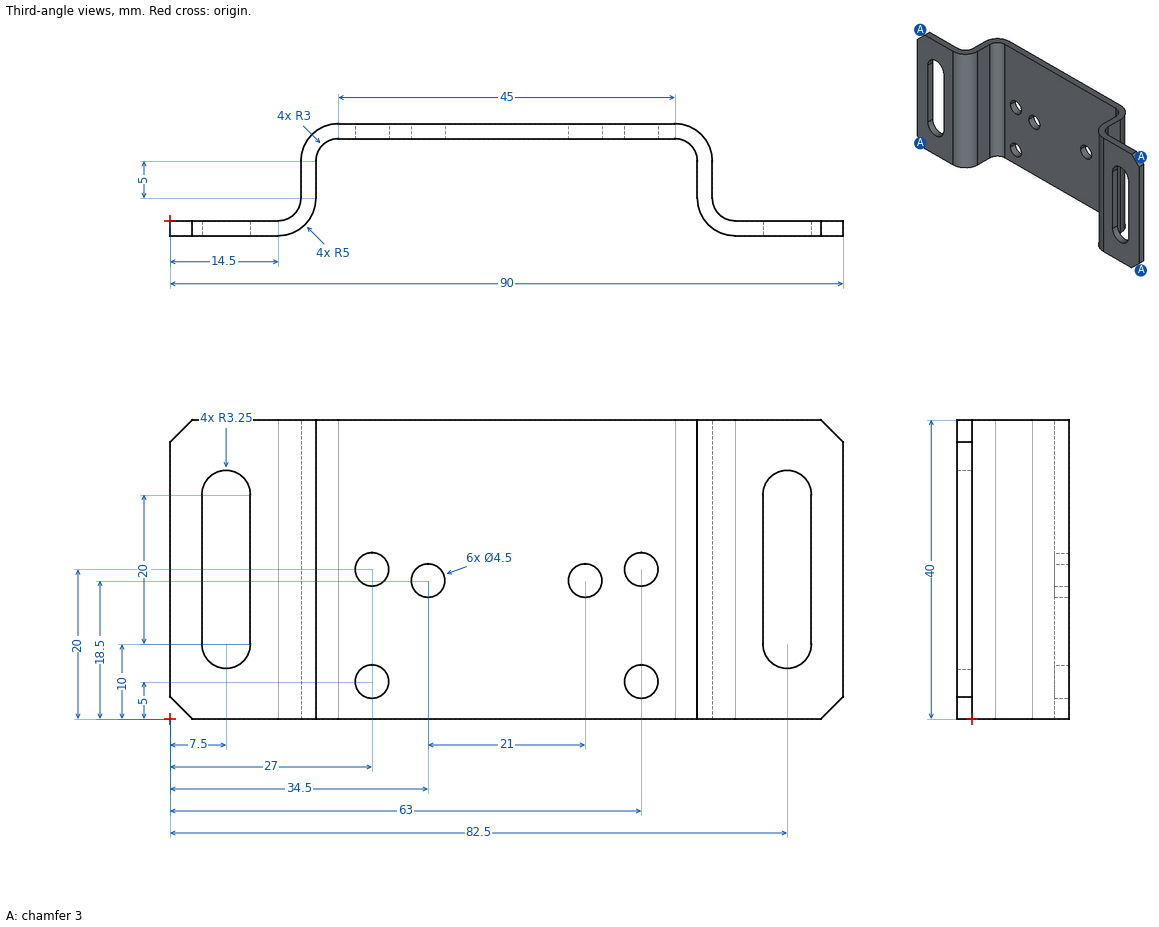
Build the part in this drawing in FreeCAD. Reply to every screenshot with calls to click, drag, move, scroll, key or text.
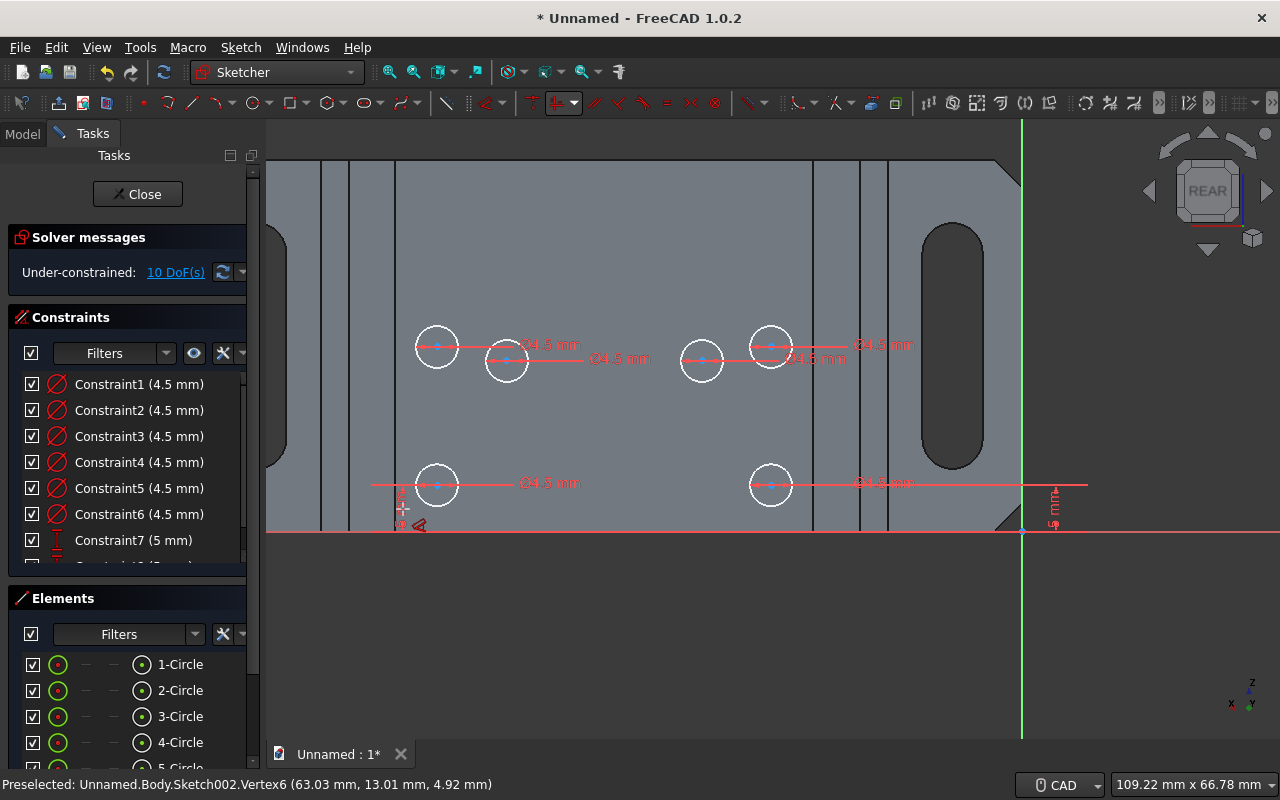
click(771, 347)
click(897, 566)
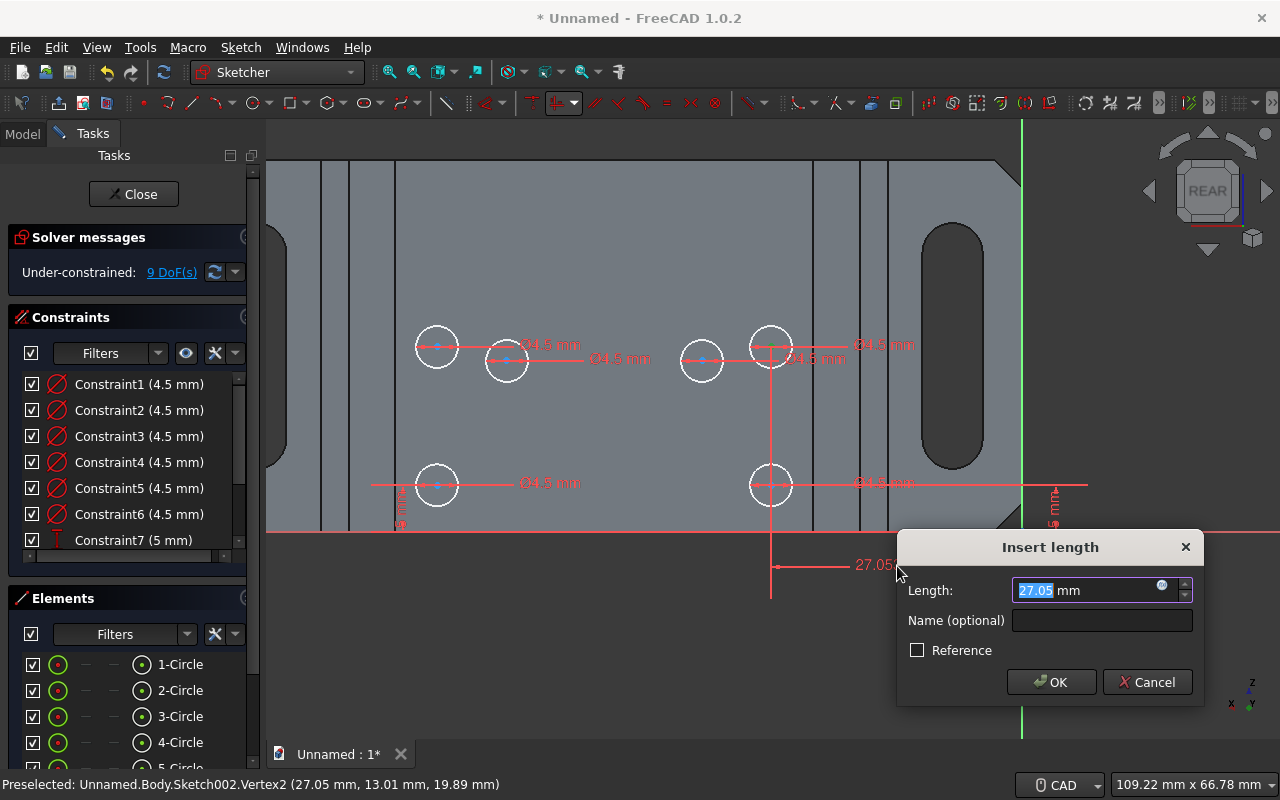
text(27)
key(Return)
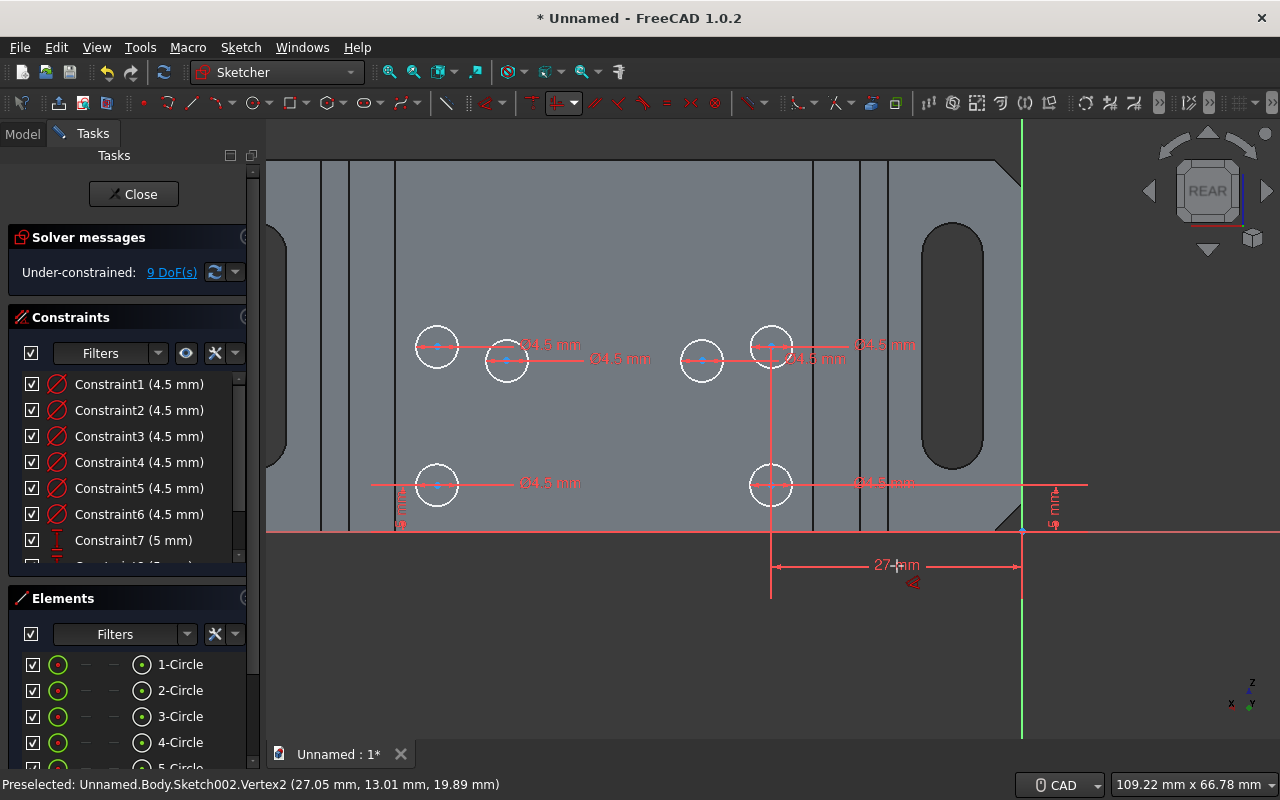
click(771, 347)
click(1056, 439)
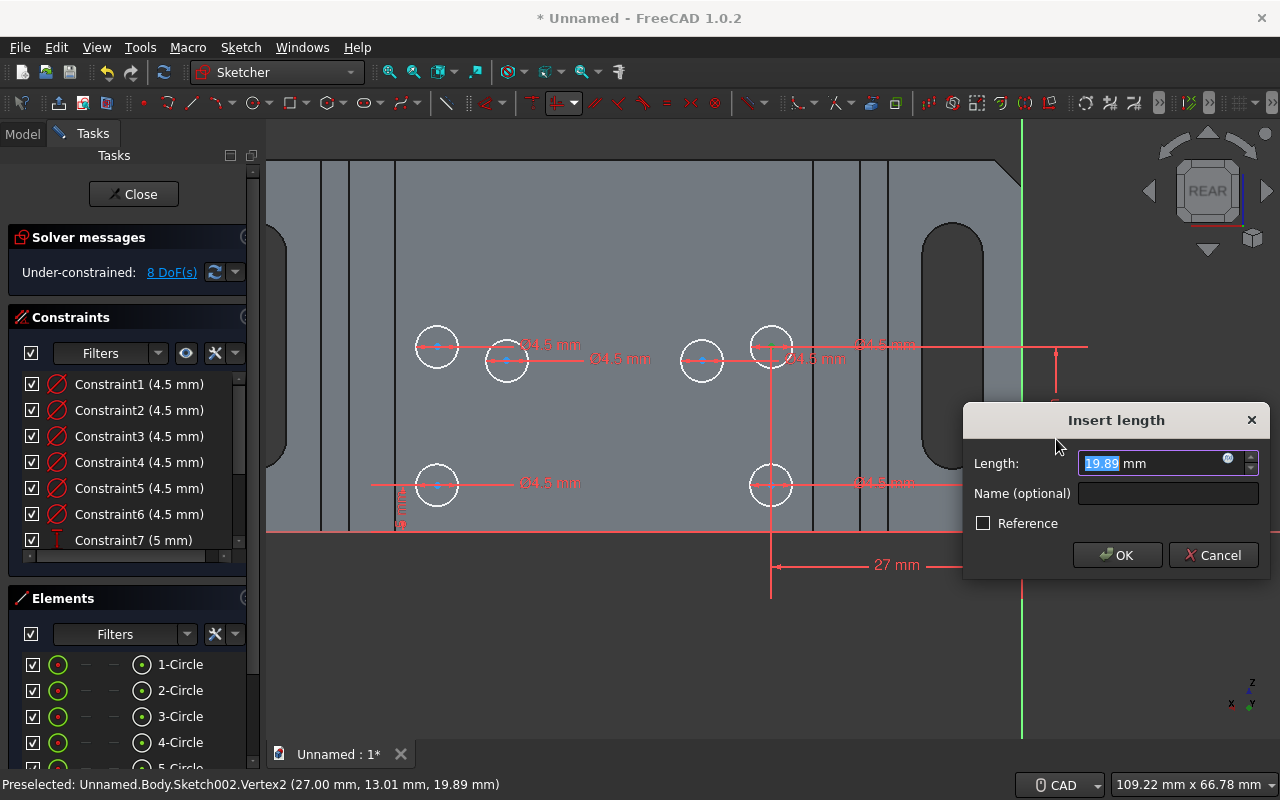
text(20)
key(Return)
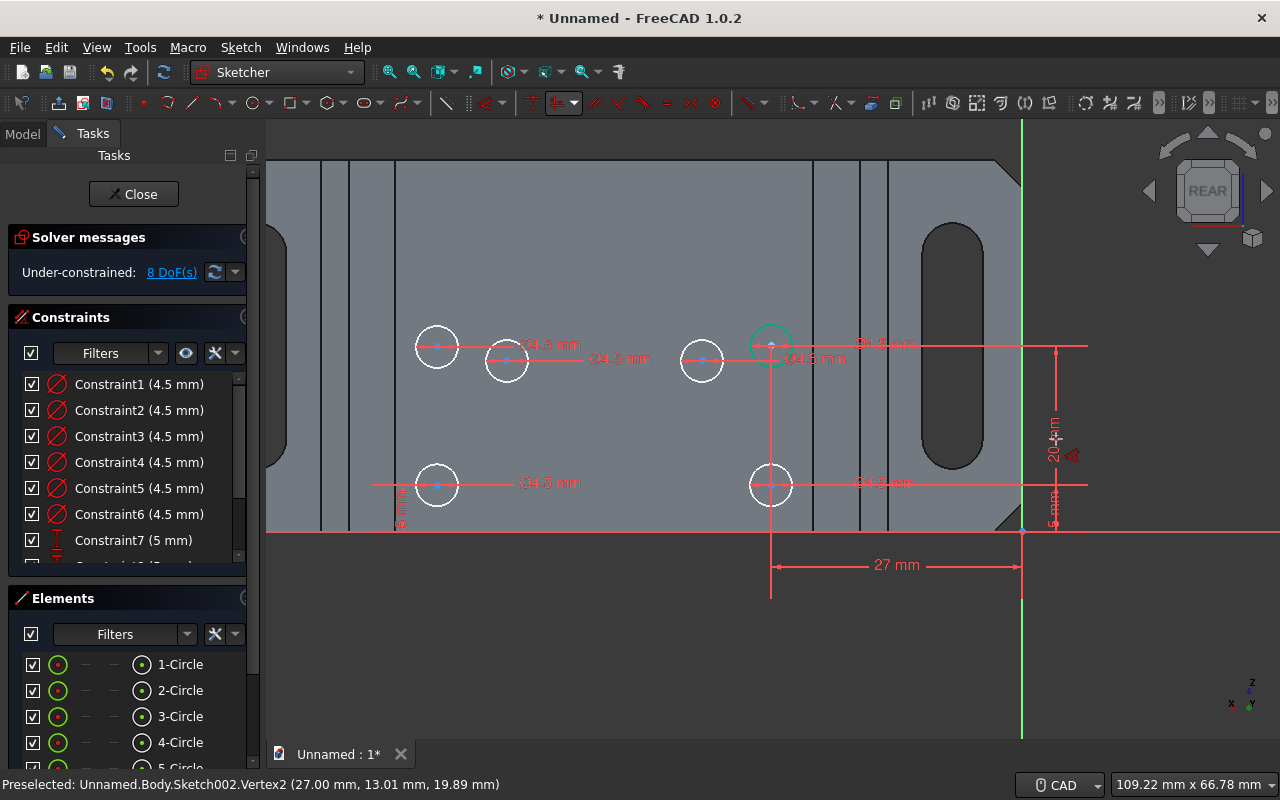
click(437, 347)
click(730, 566)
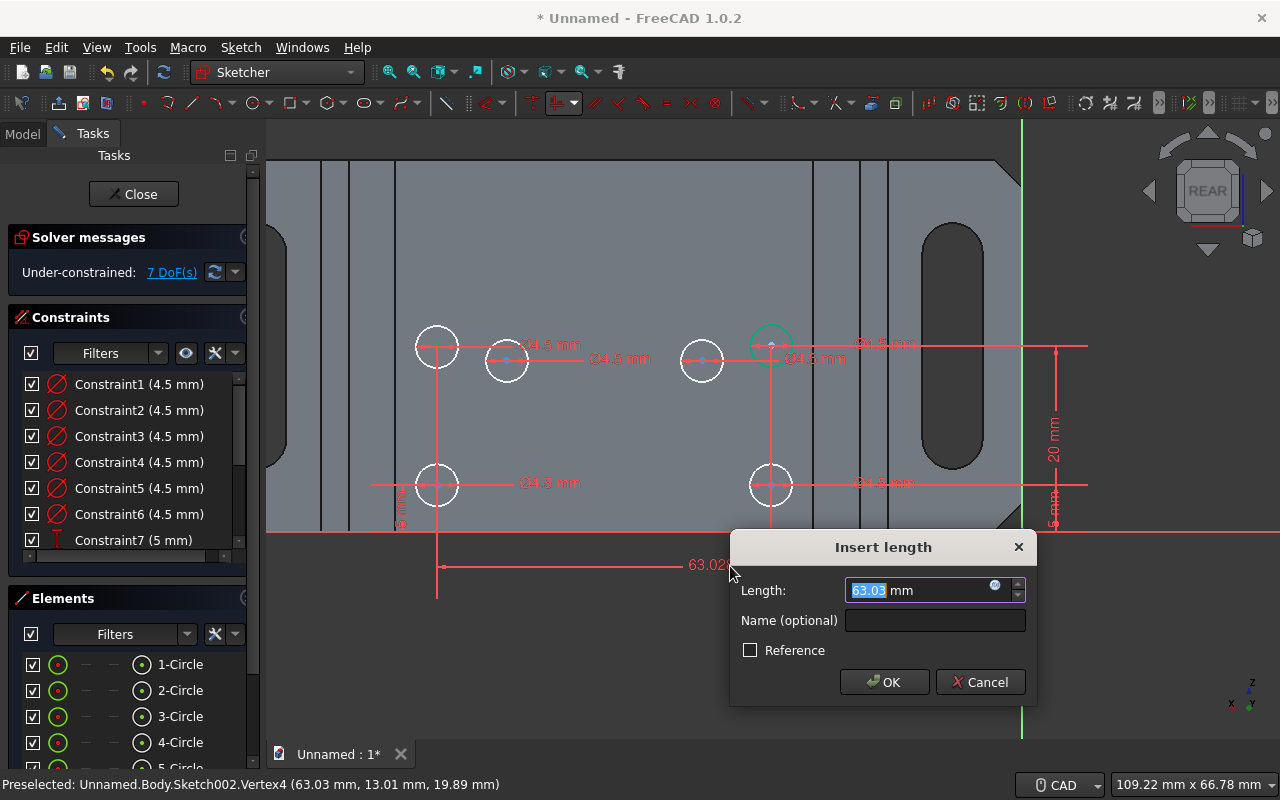
text(63)
key(Return)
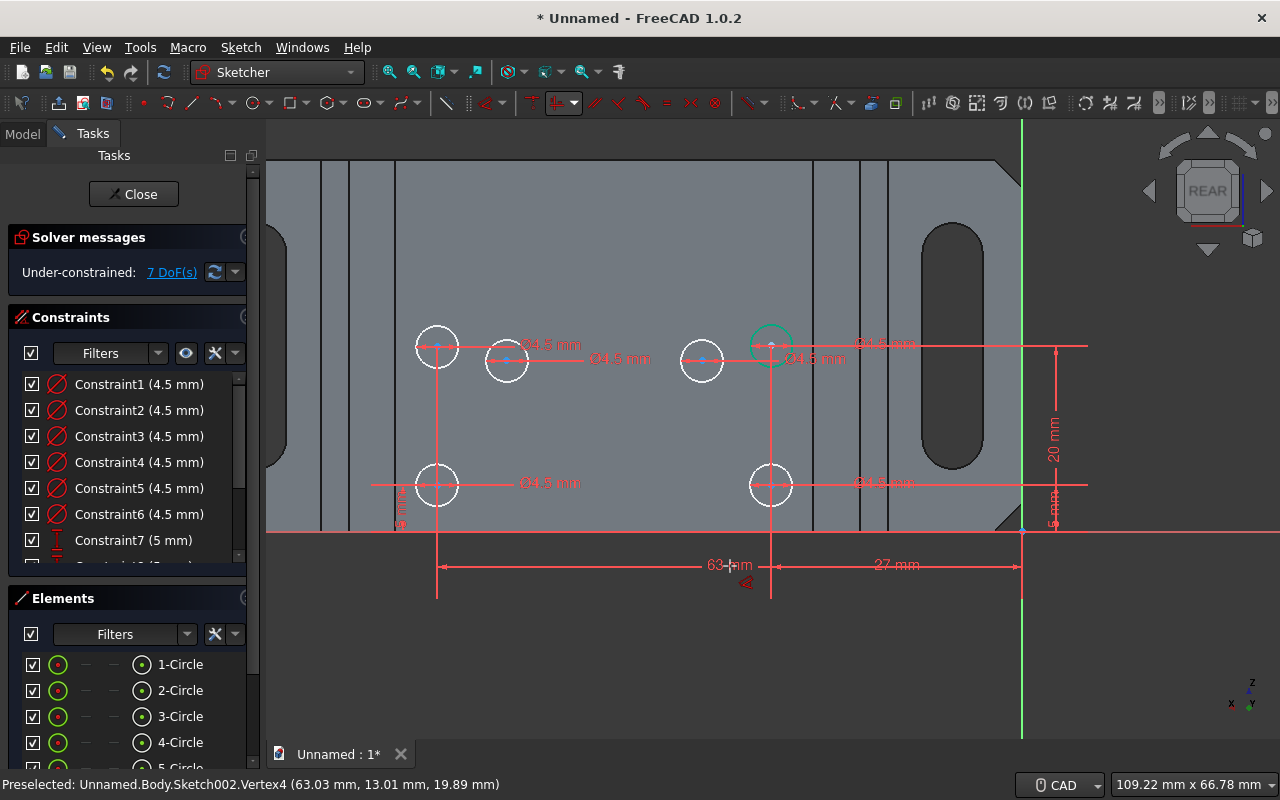
click(437, 347)
click(1056, 397)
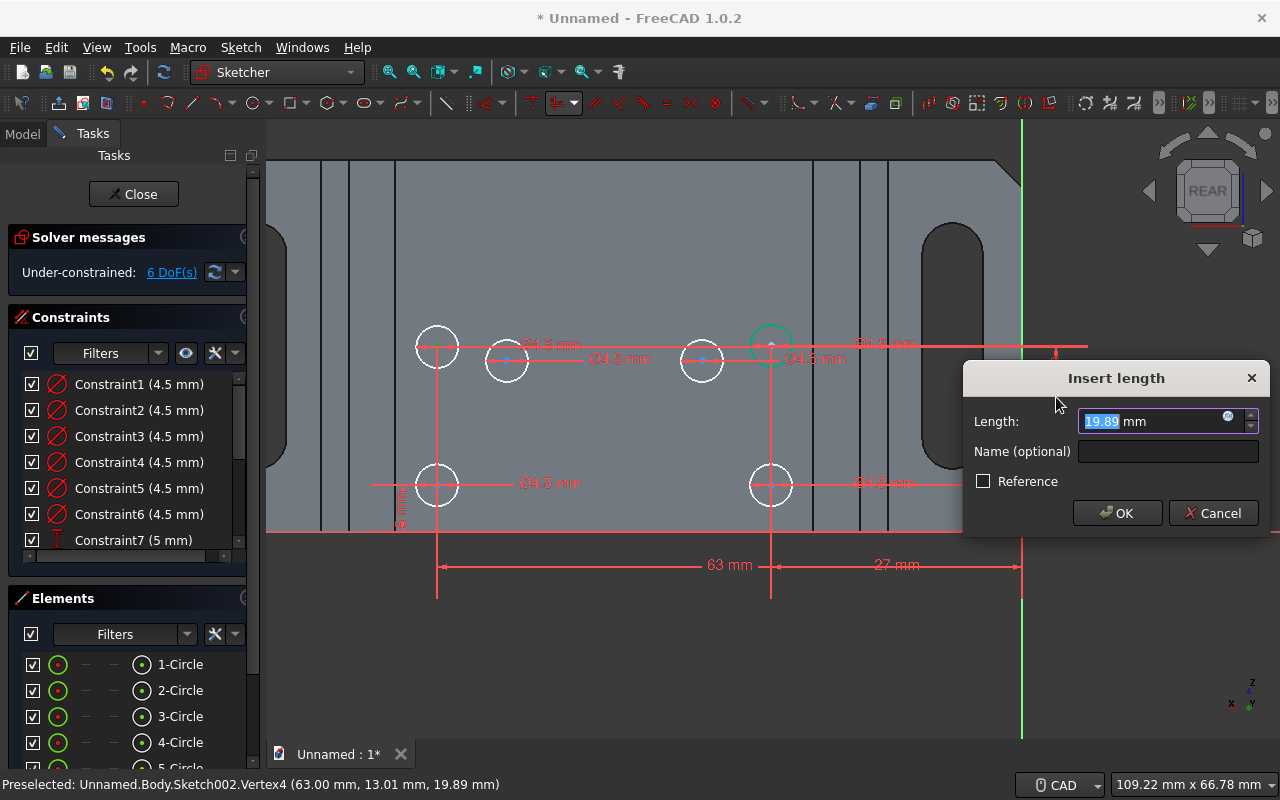
text(20)
key(Return)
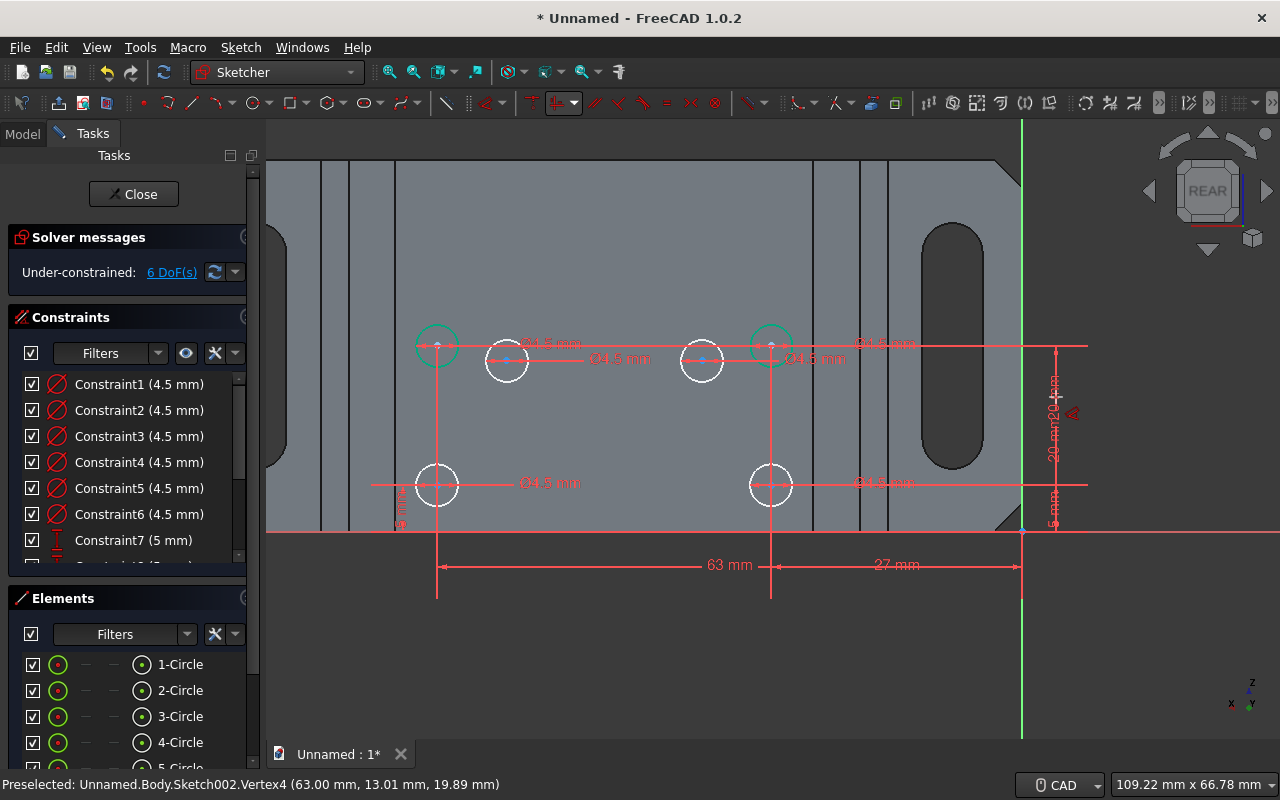
click(771, 485)
click(809, 566)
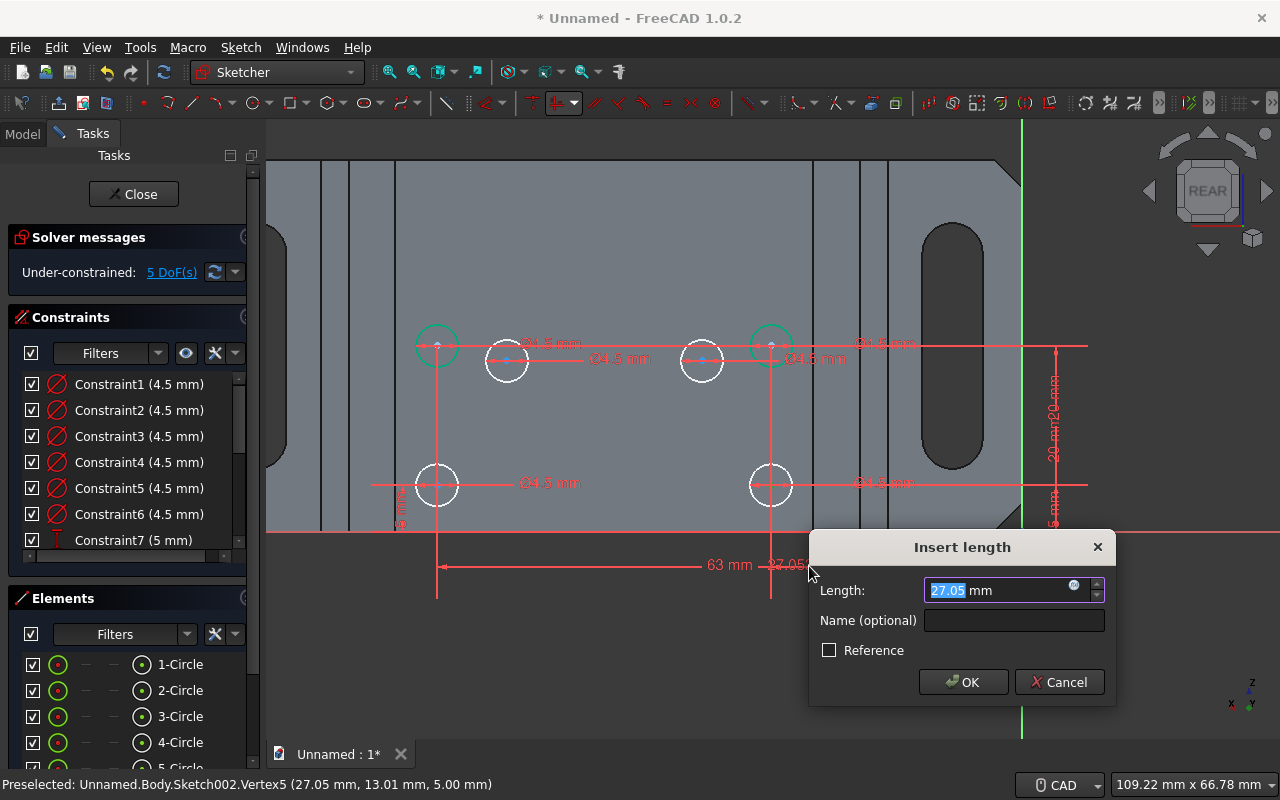
text(27)
key(Return)